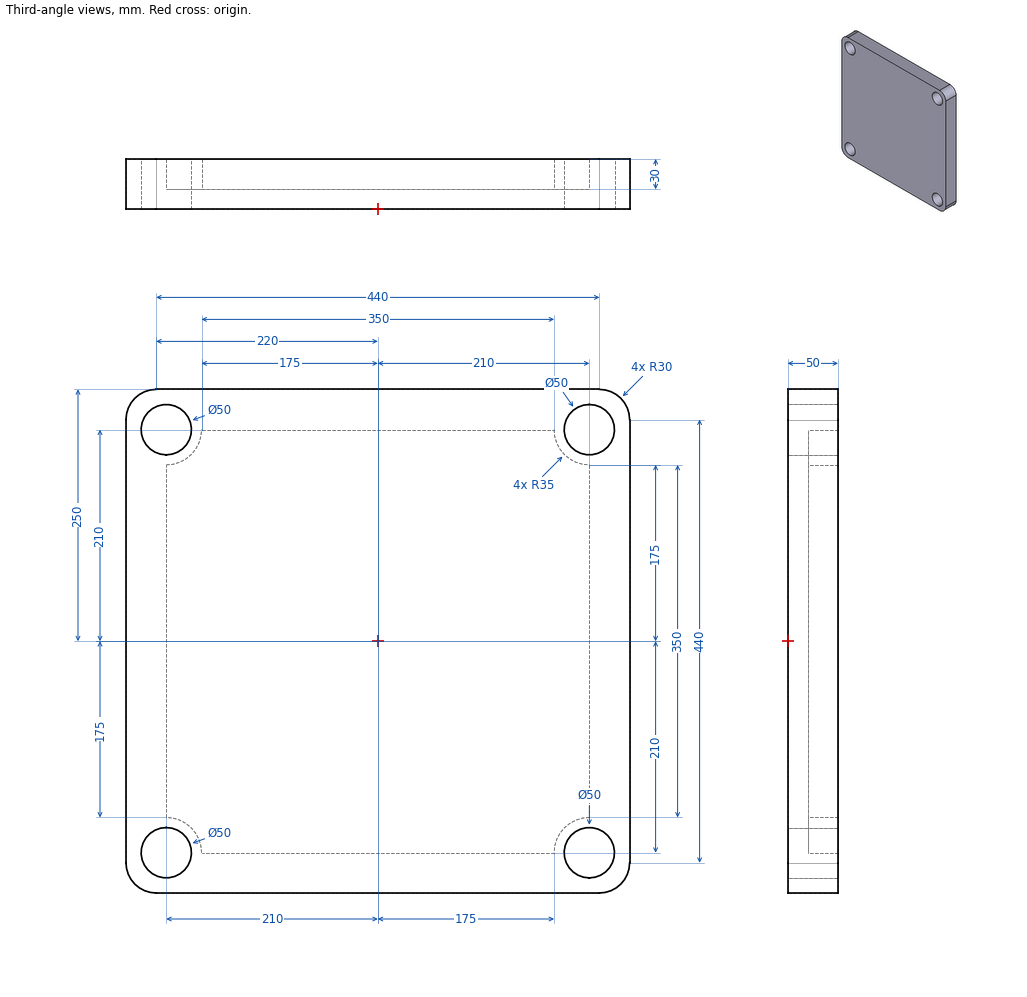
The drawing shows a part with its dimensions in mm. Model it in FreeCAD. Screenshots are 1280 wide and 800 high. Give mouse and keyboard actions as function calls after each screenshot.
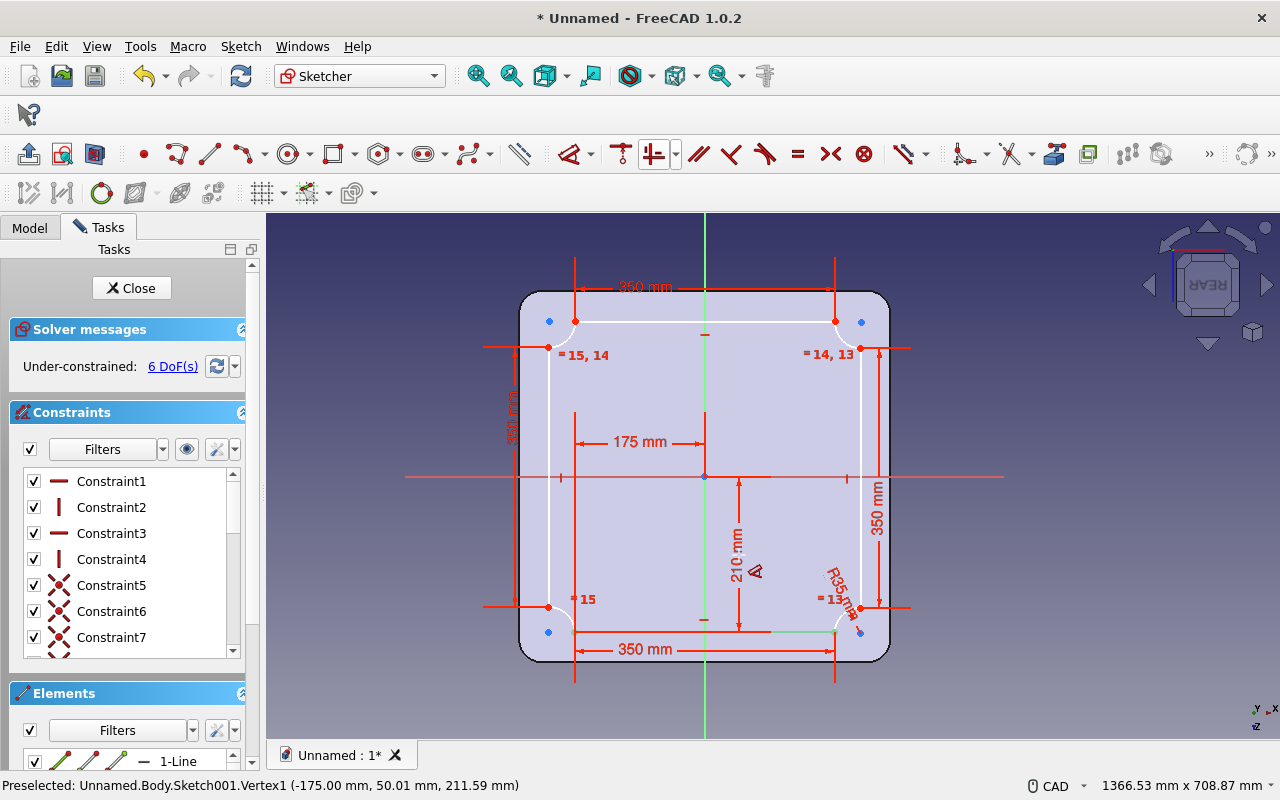
click(861, 608)
click(783, 443)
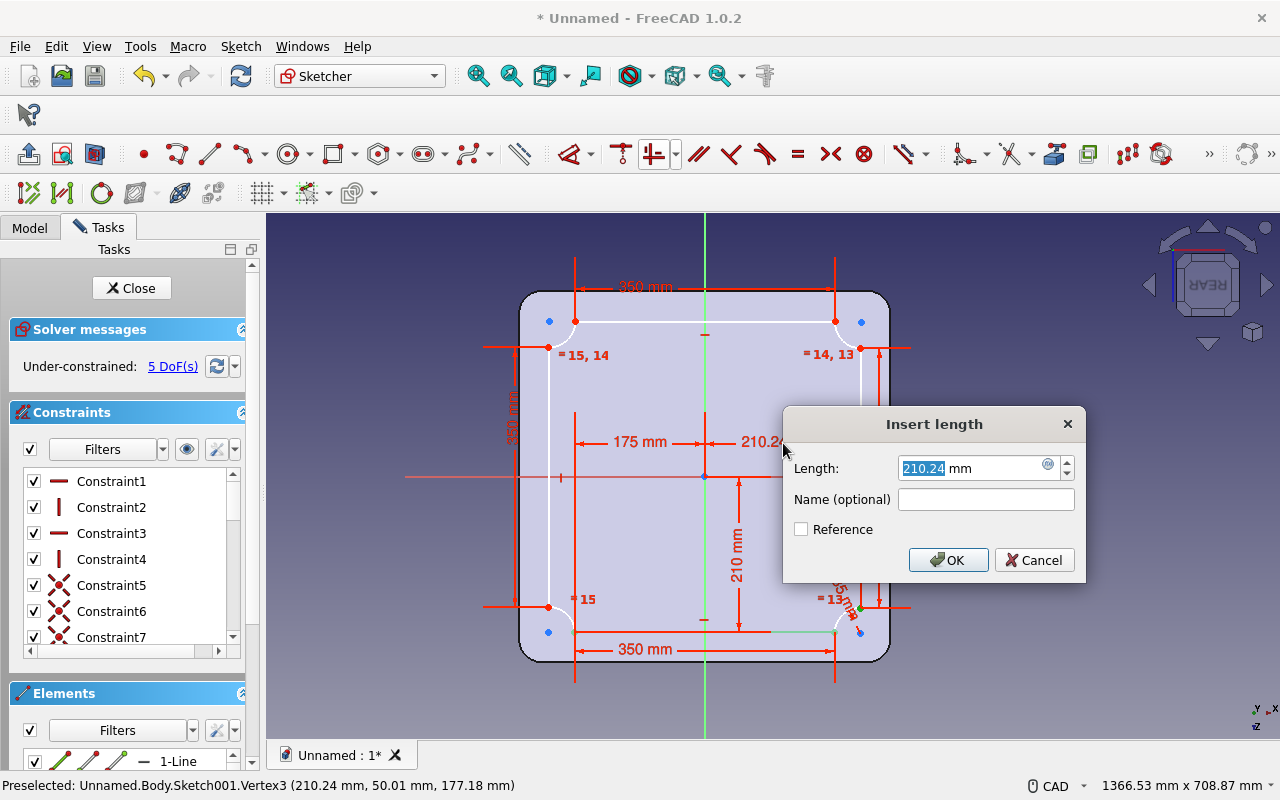
text(210)
key(Return)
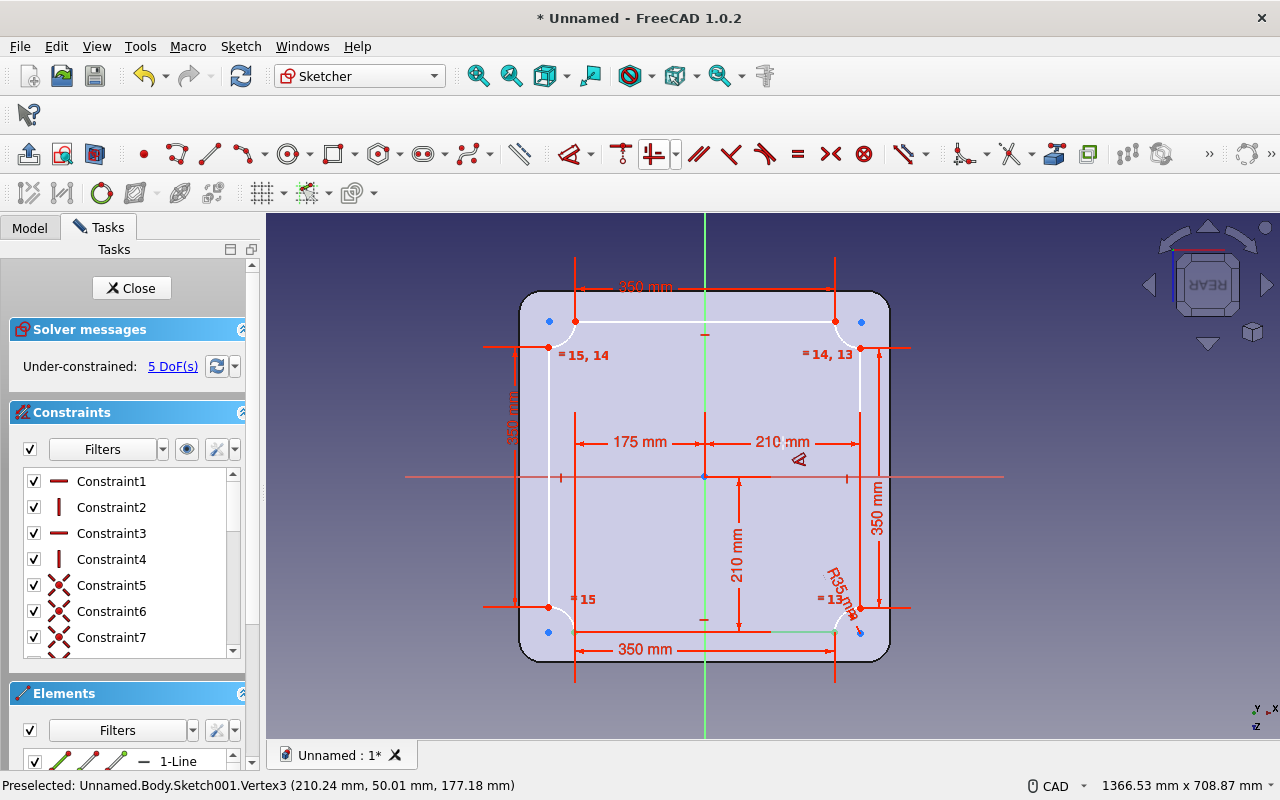
click(860, 608)
click(894, 542)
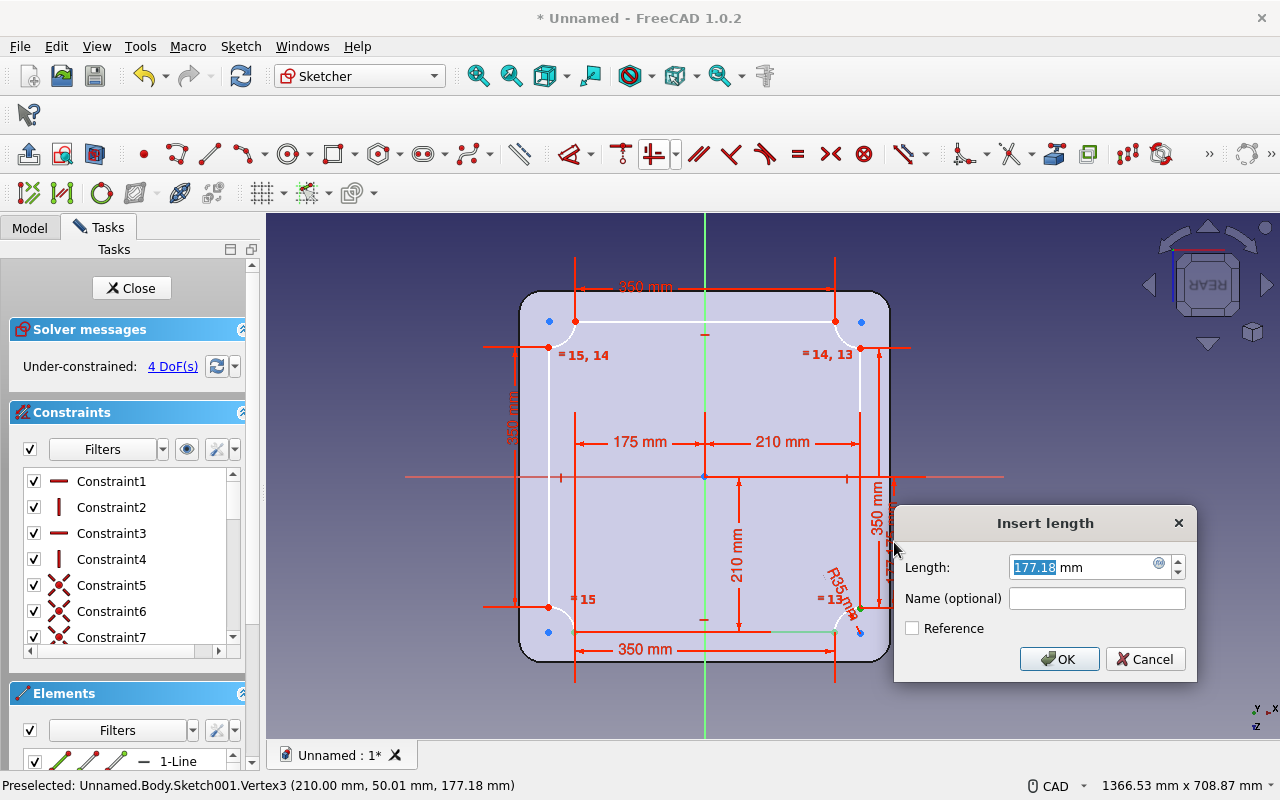
text(175)
key(Return)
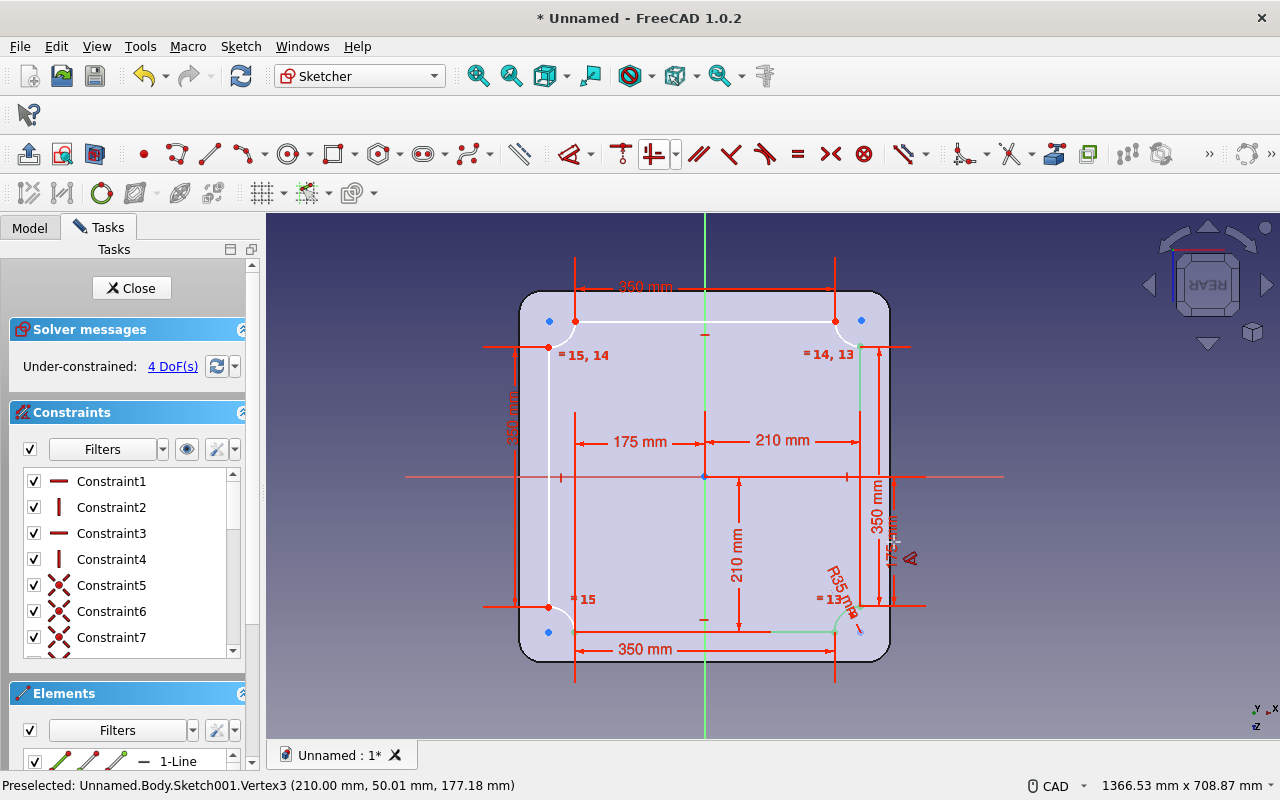
click(835, 322)
click(770, 288)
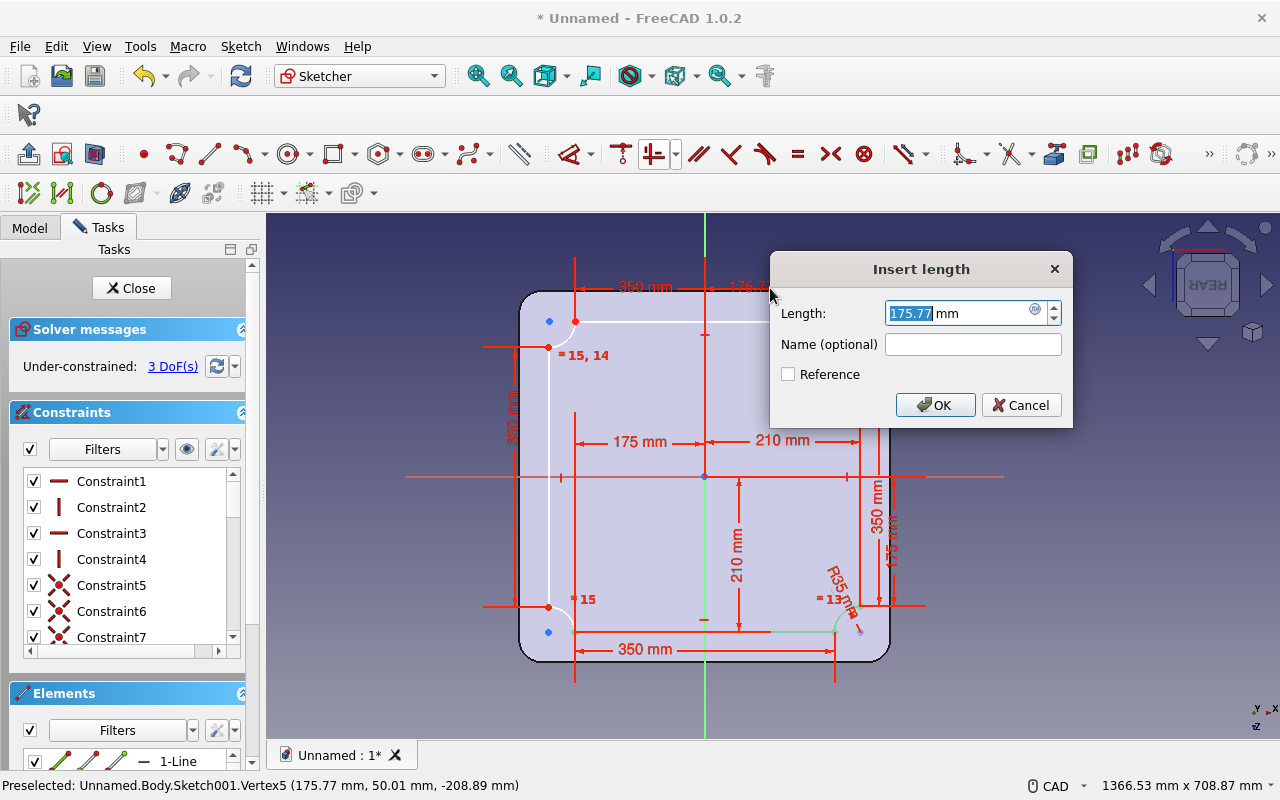
text(175)
key(Return)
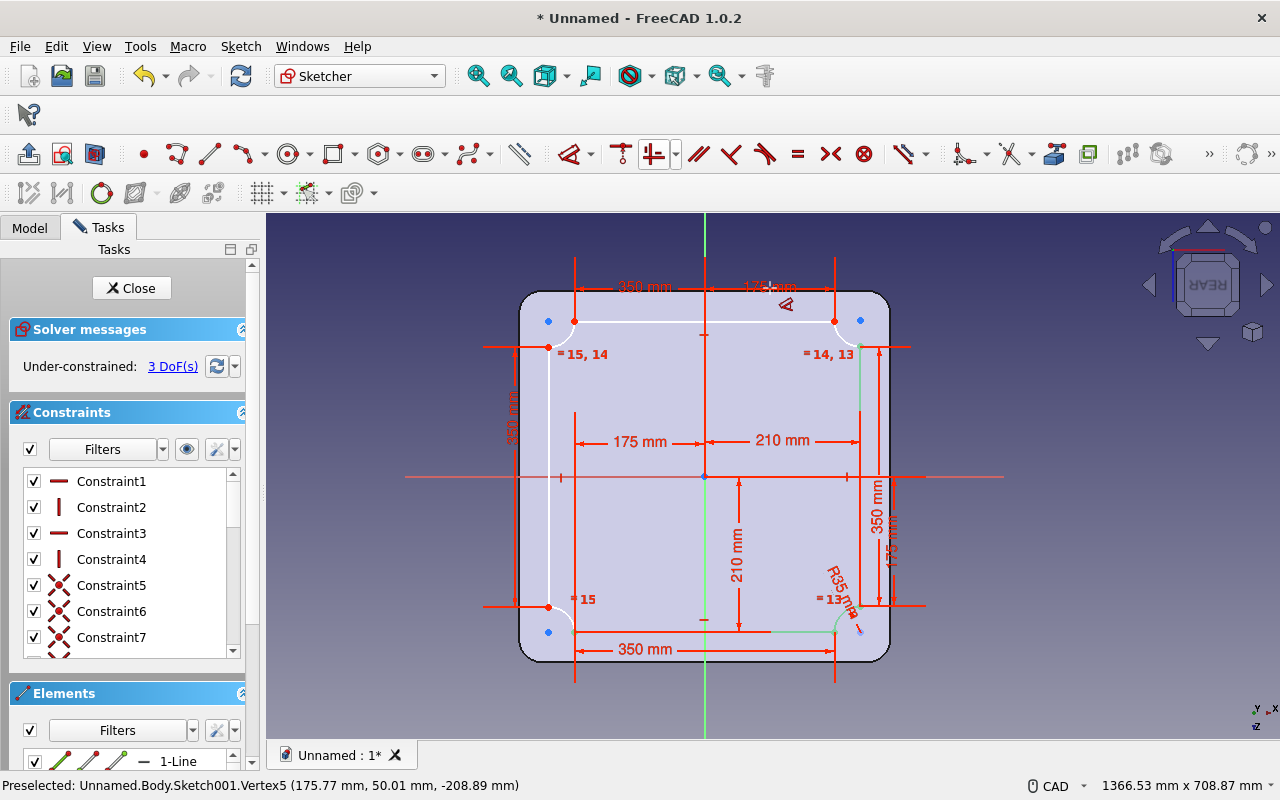
click(835, 322)
click(671, 399)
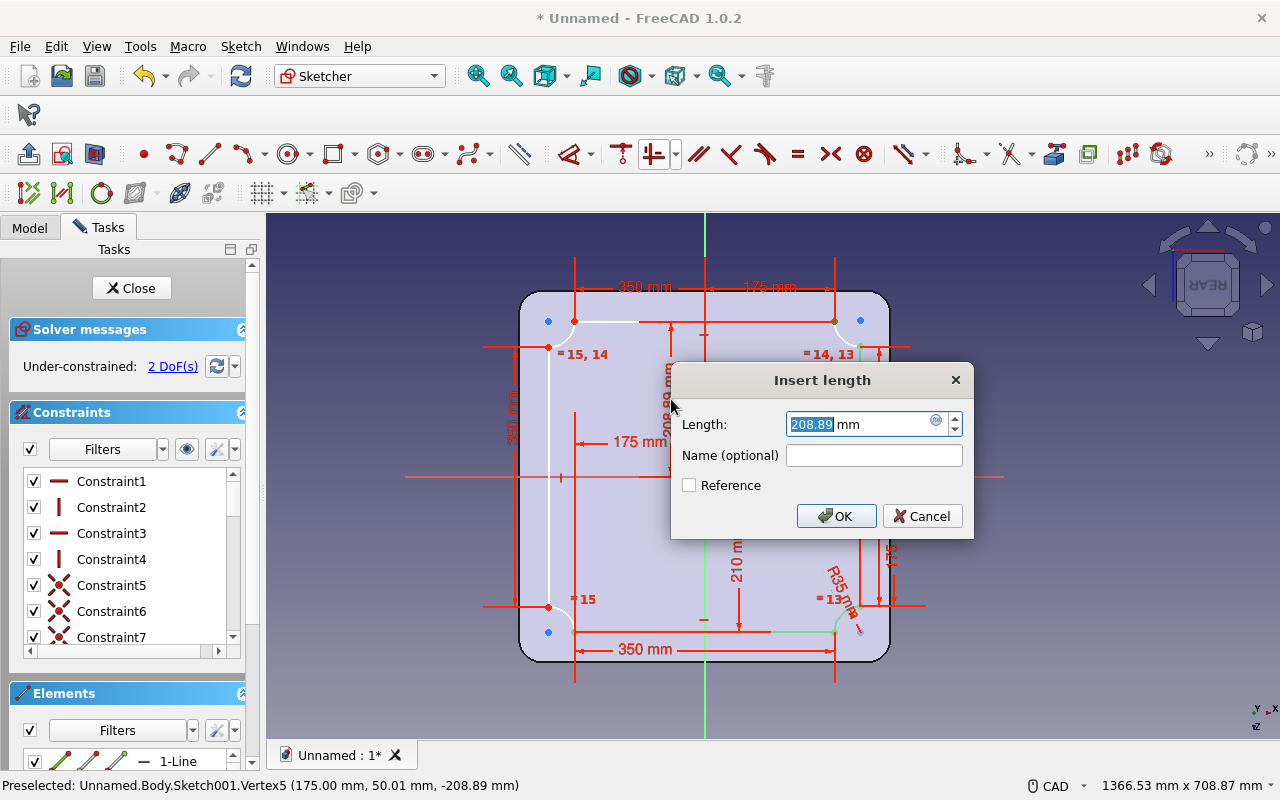
text(210)
key(Return)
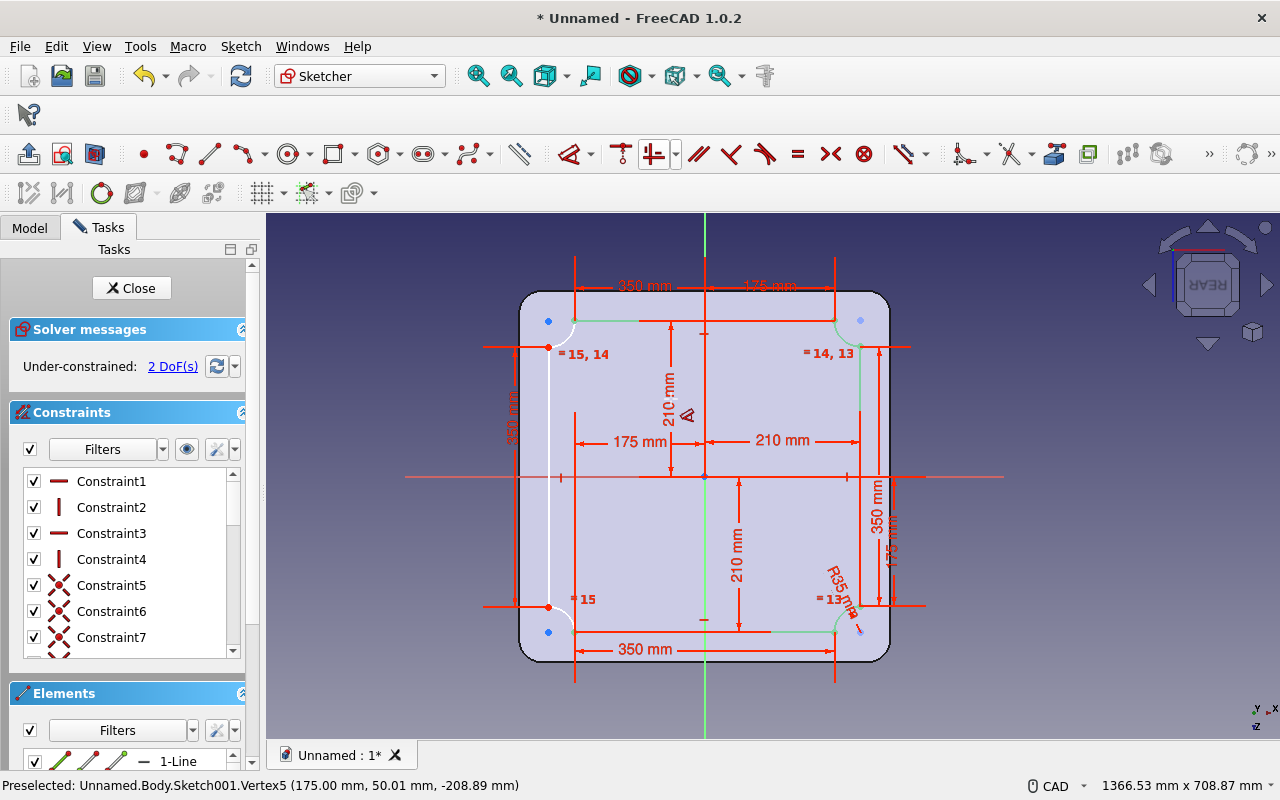
click(549, 347)
click(627, 511)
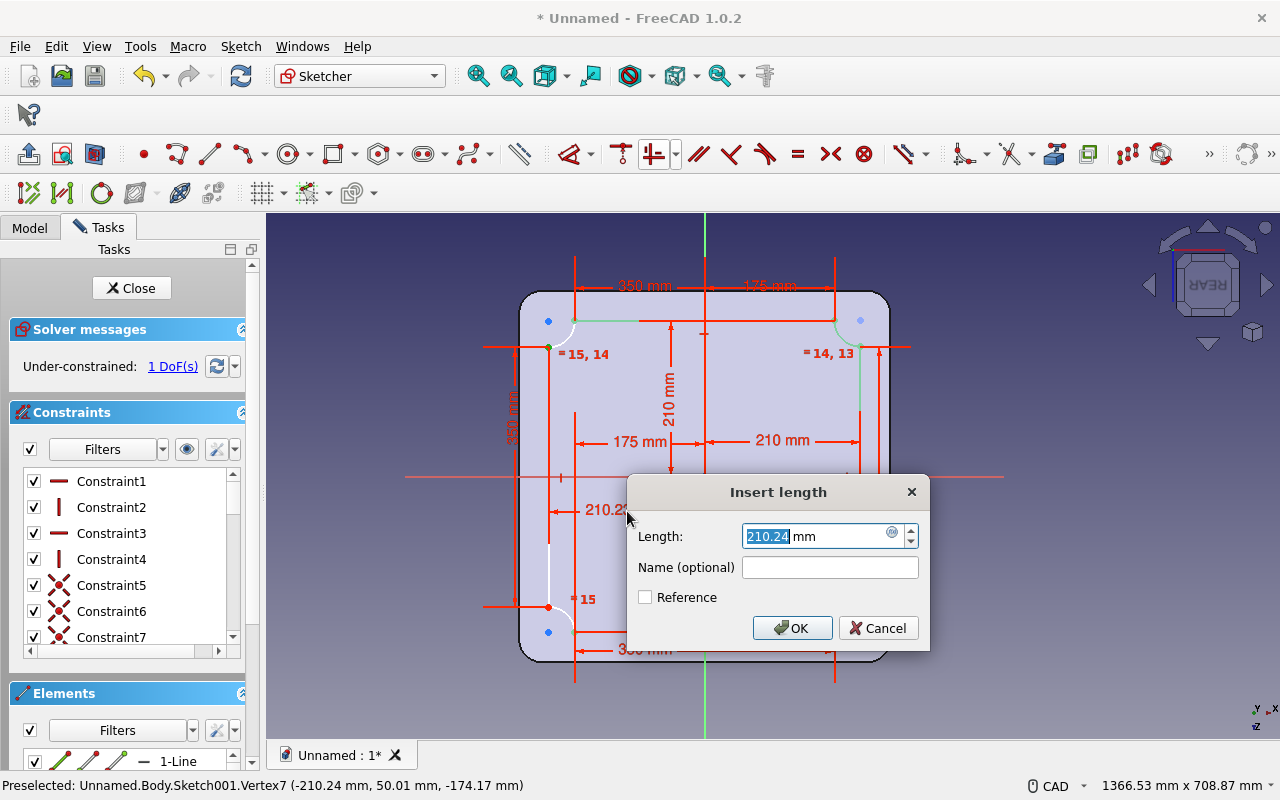
text(210)
key(Return)